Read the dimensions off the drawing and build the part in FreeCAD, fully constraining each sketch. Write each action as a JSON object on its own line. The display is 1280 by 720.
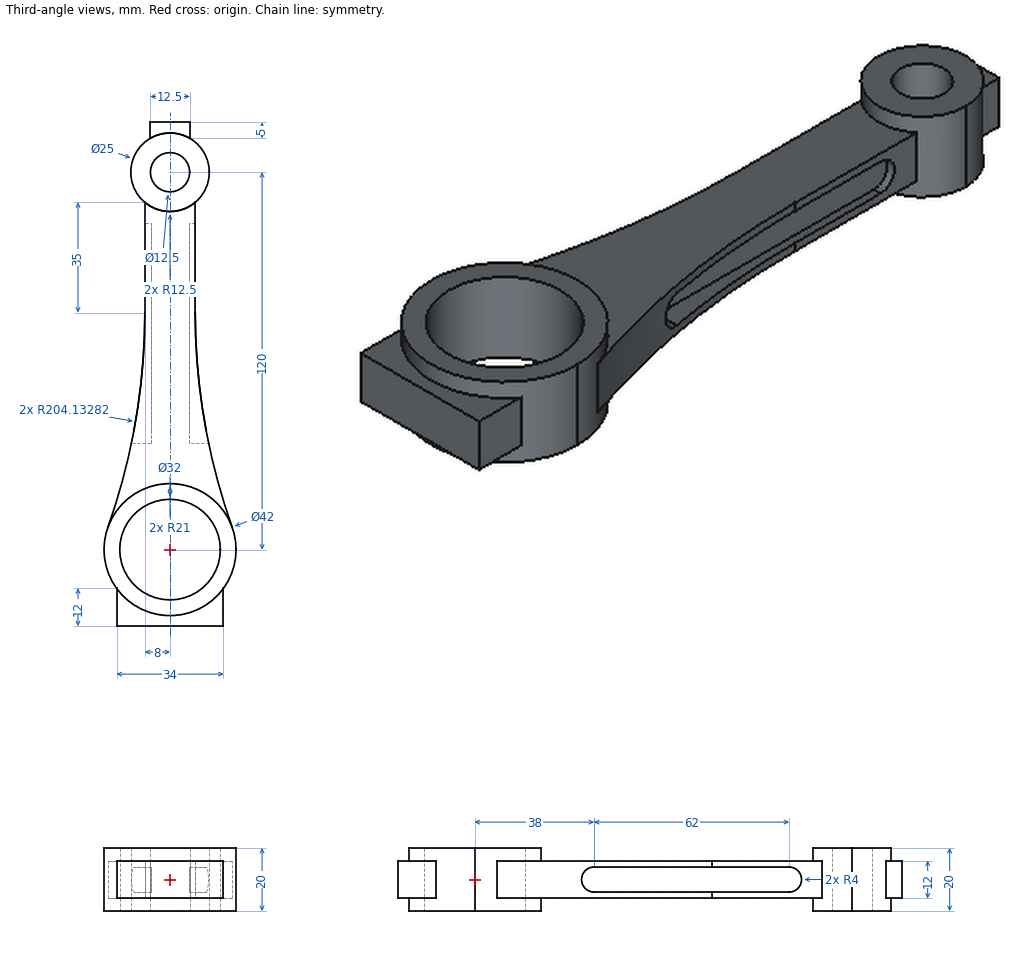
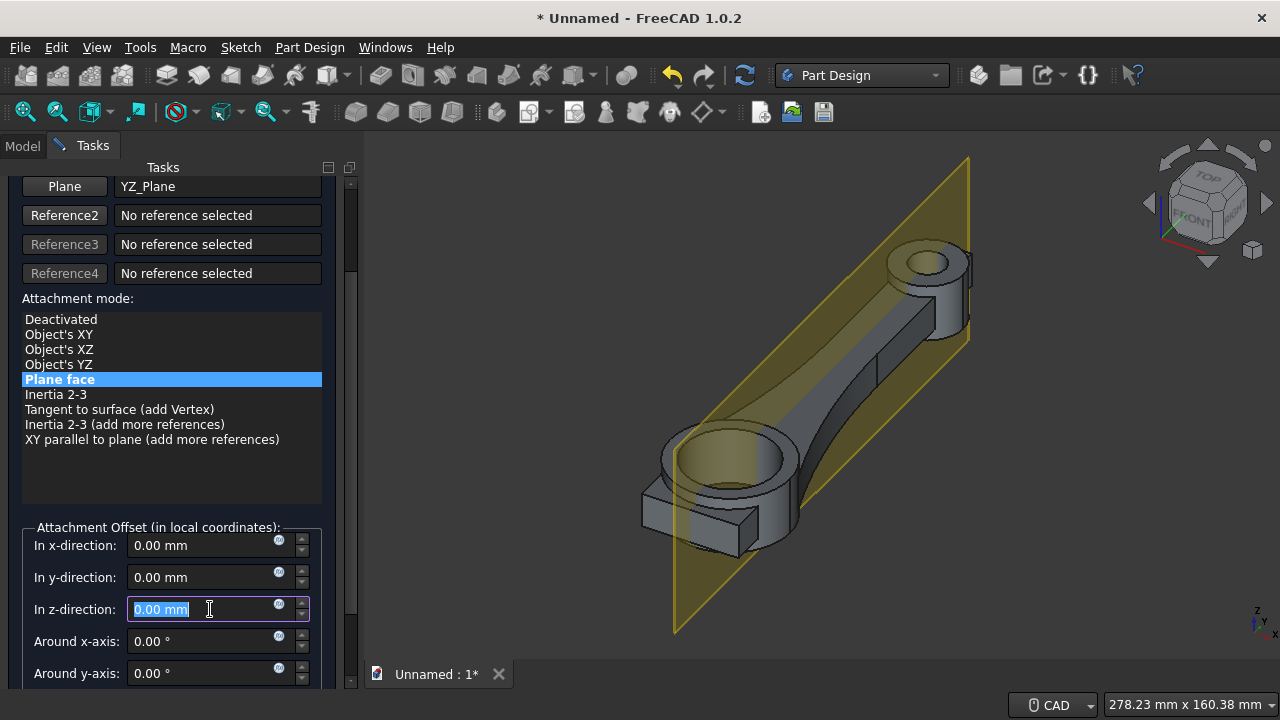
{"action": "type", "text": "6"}
{"action": "key", "text": "Tab"}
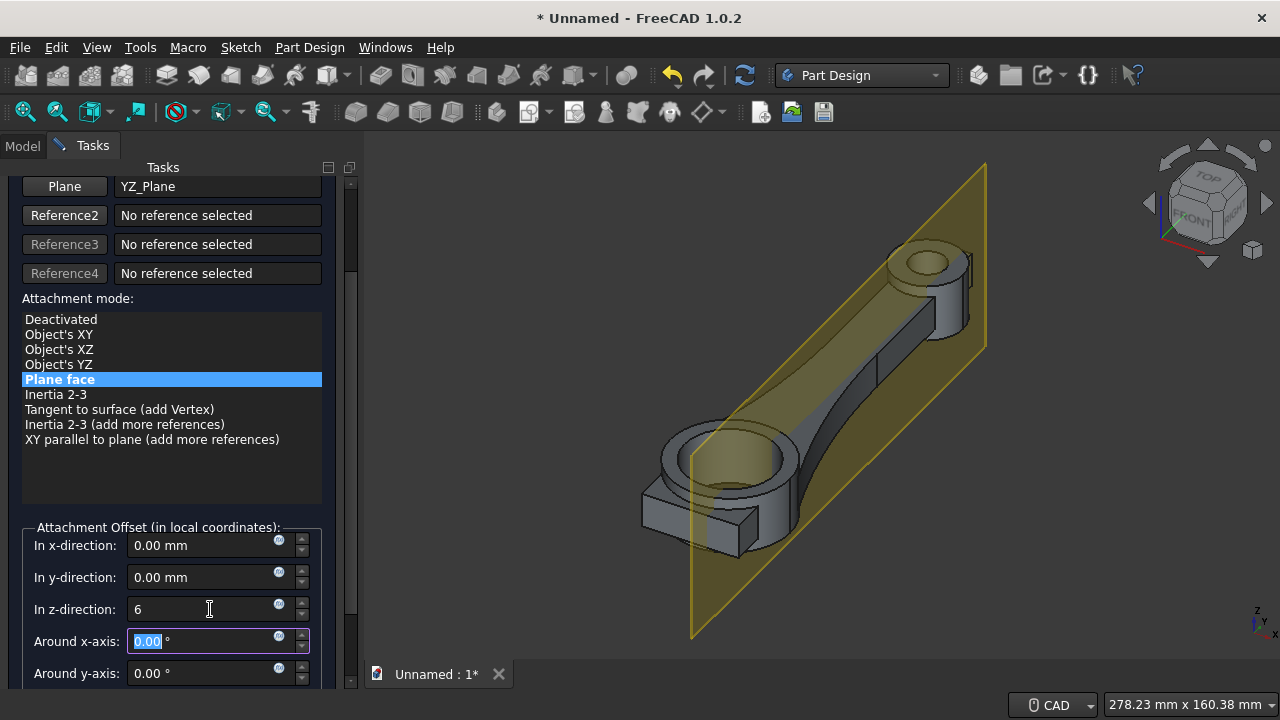
{"action": "scroll", "coordinate": [351, 432], "scroll_direction": "up", "scroll_amount": 3}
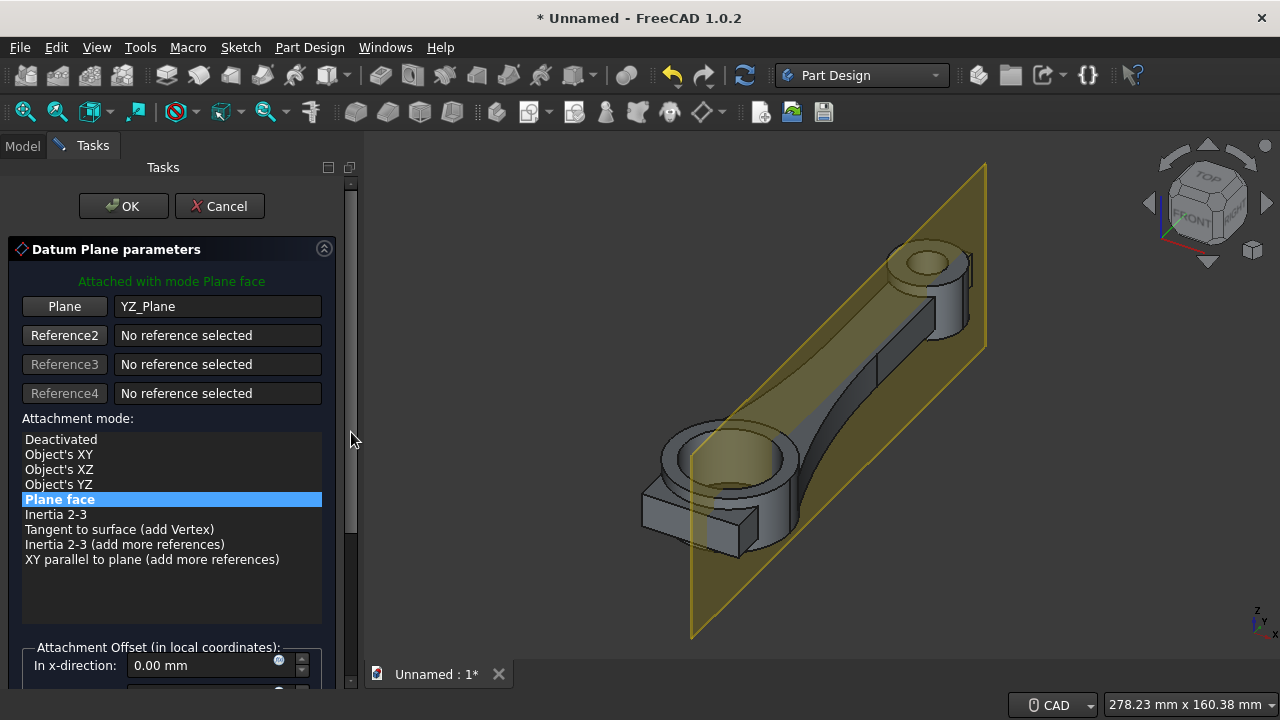
{"action": "left_click", "coordinate": [124, 206]}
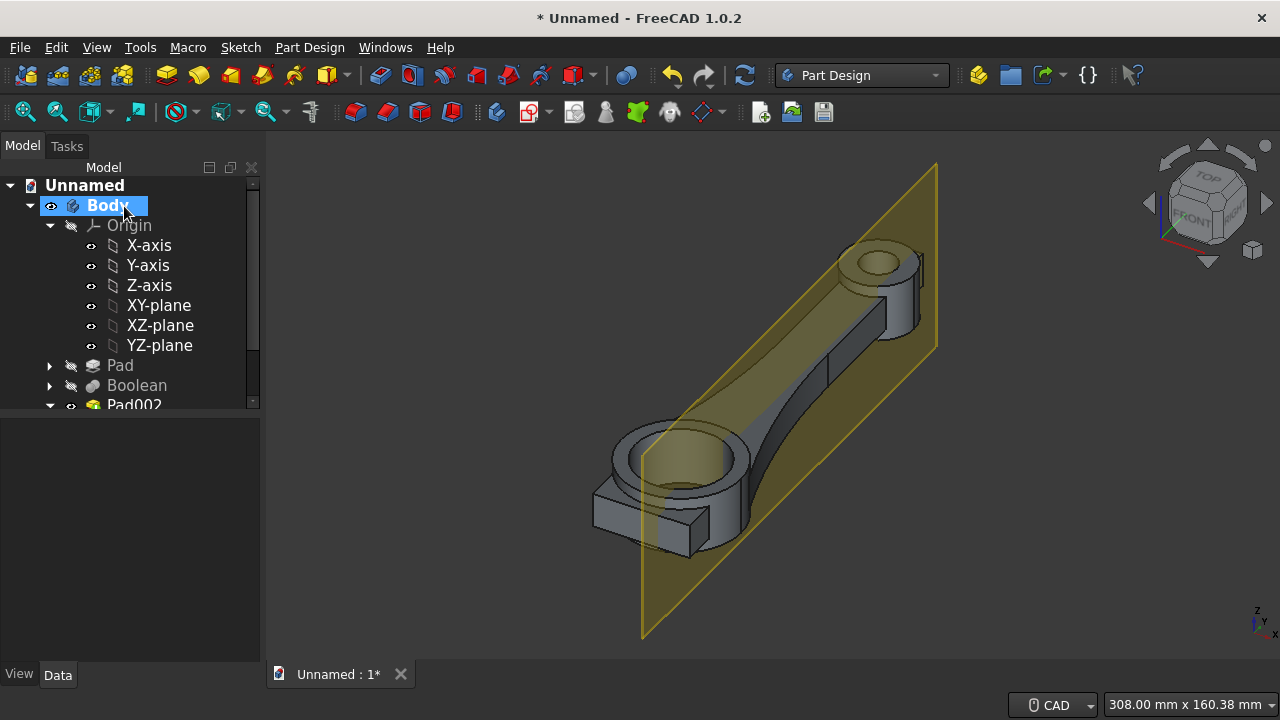
{"action": "scroll", "coordinate": [100, 301], "scroll_direction": "down", "scroll_amount": 3}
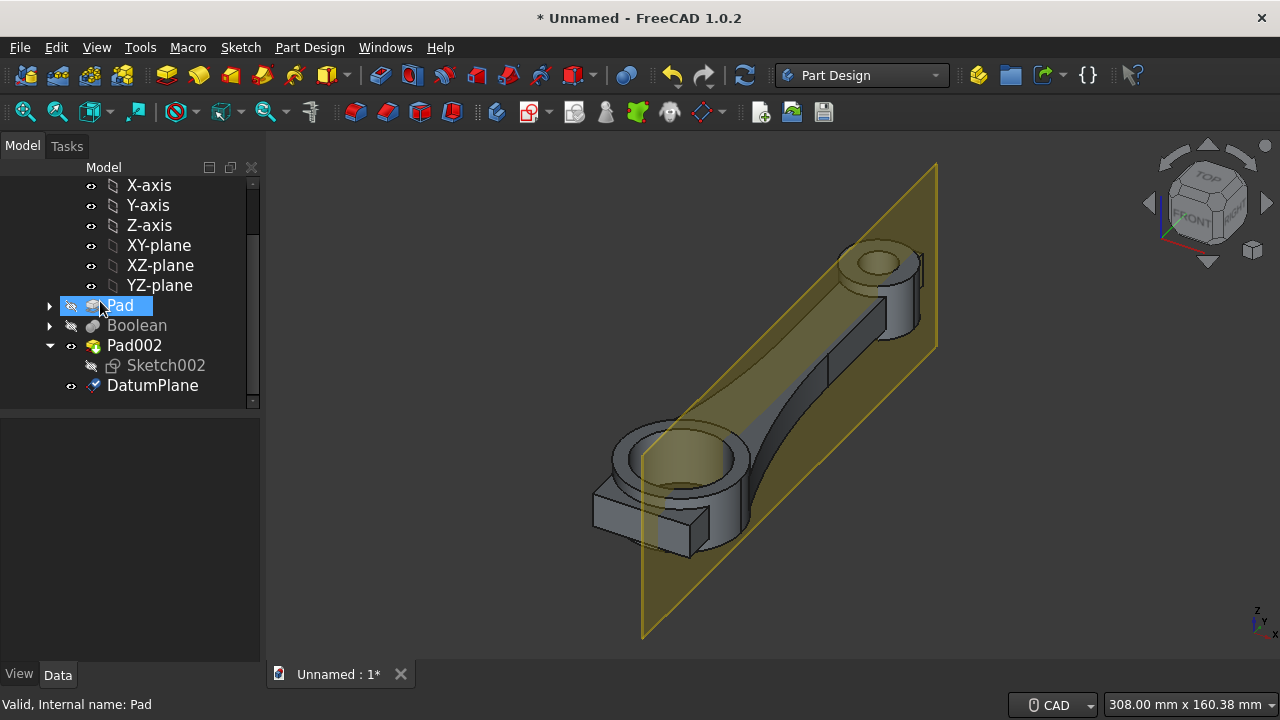
{"action": "left_click", "coordinate": [116, 386]}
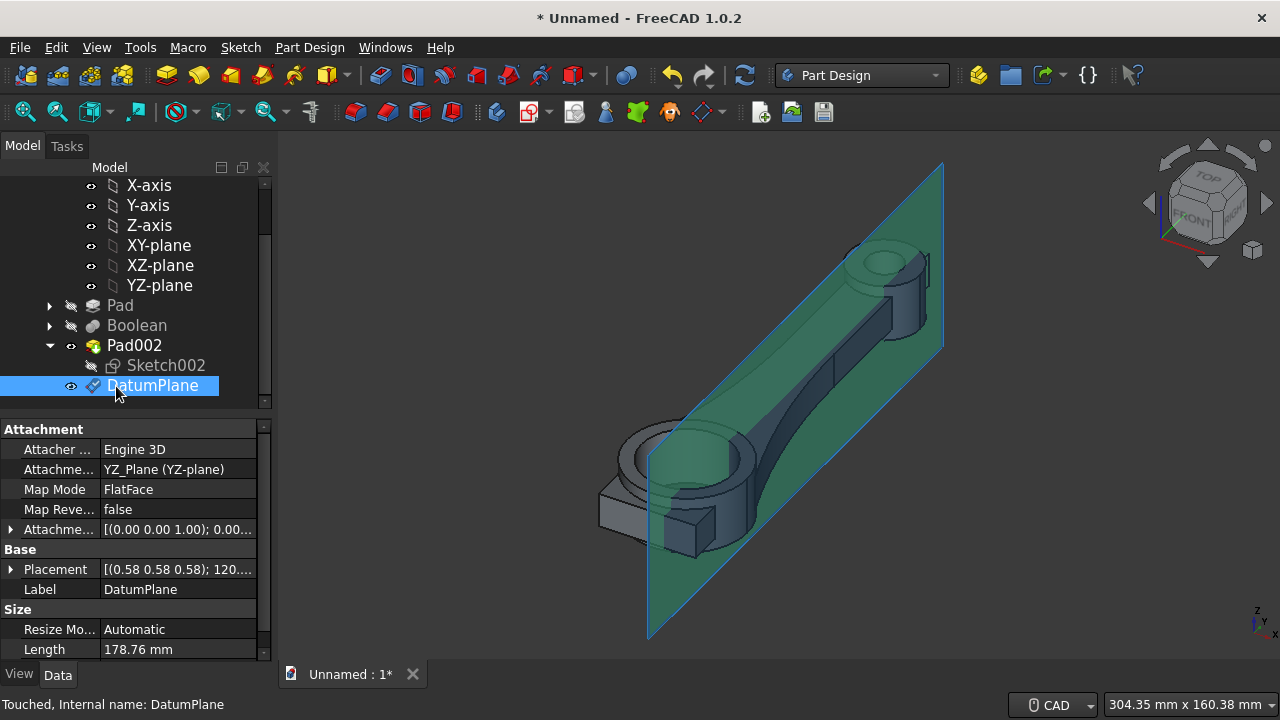
{"action": "left_click", "coordinate": [530, 112]}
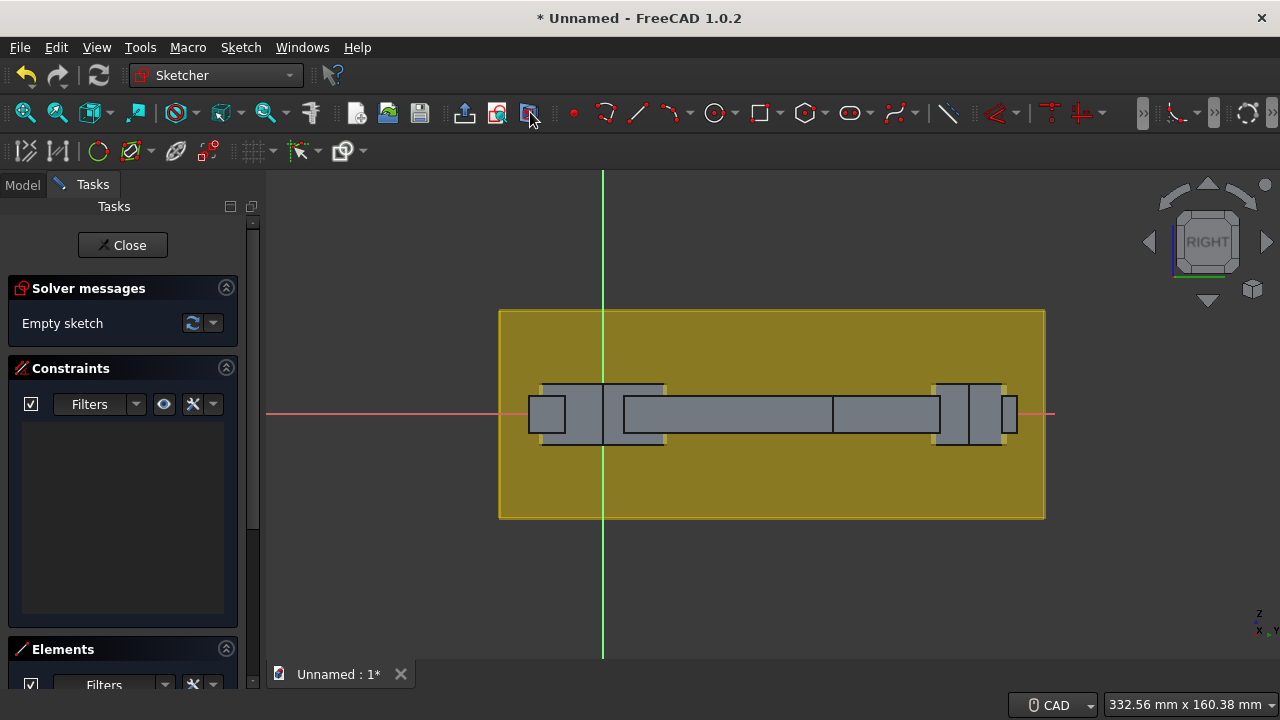
{"action": "key", "text": "q s"}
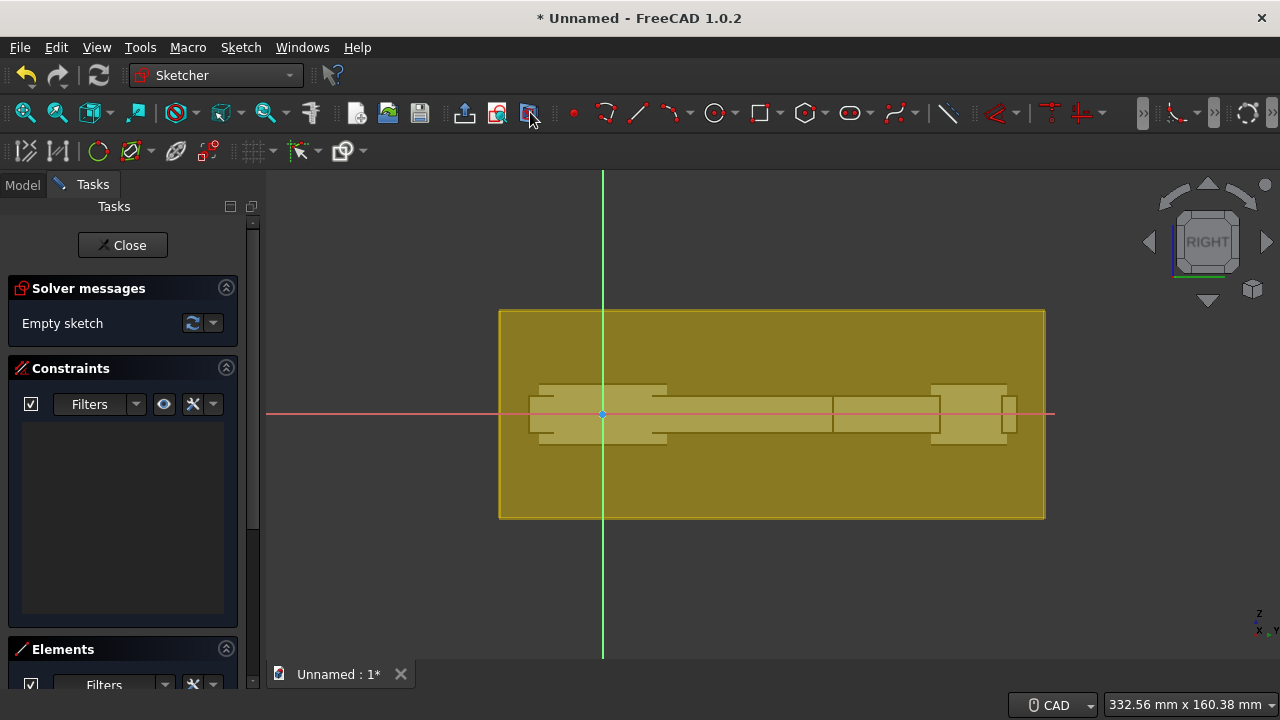
{"action": "scroll", "coordinate": [831, 414], "scroll_direction": "up", "scroll_amount": 3}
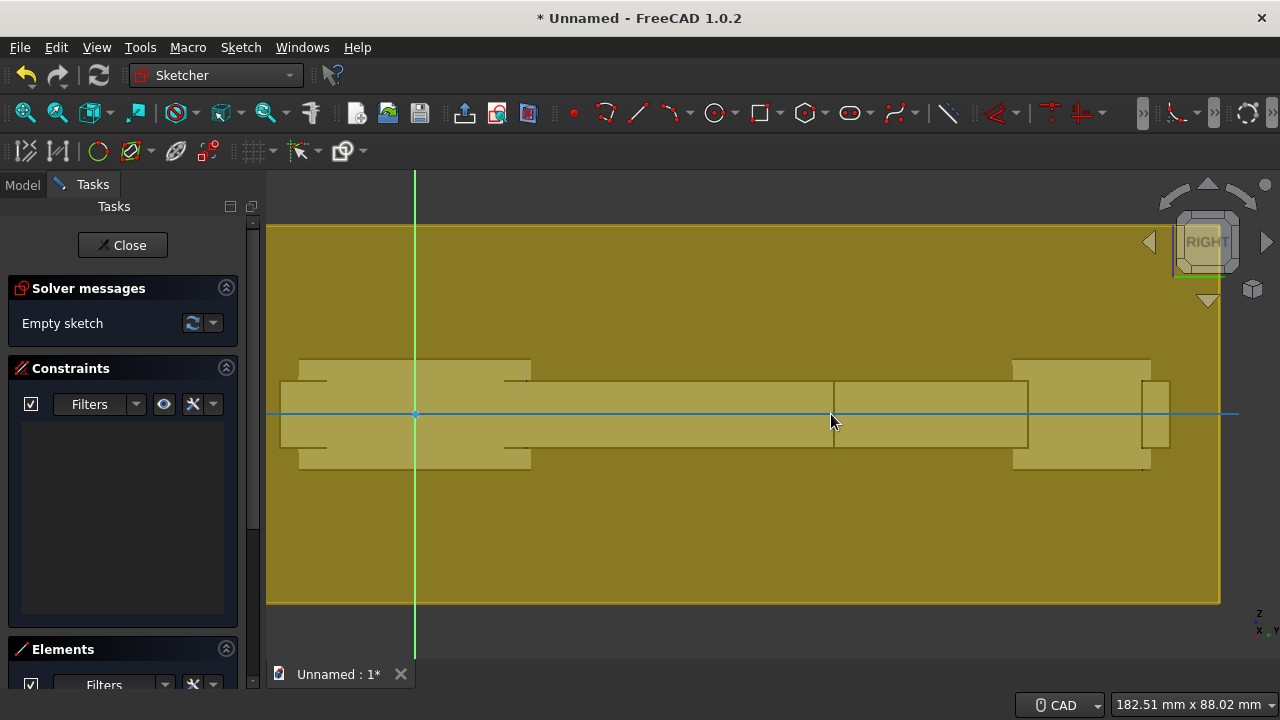
{"action": "key", "text": "g s"}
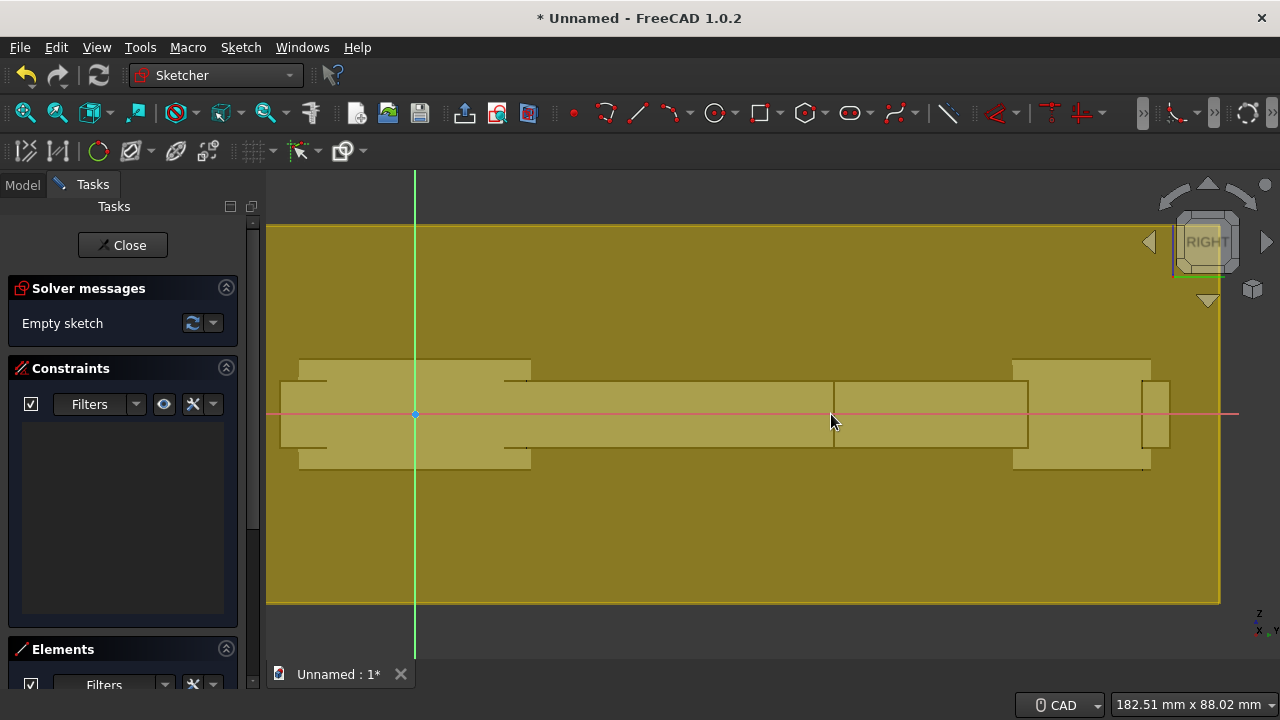
{"action": "left_click", "coordinate": [626, 414]}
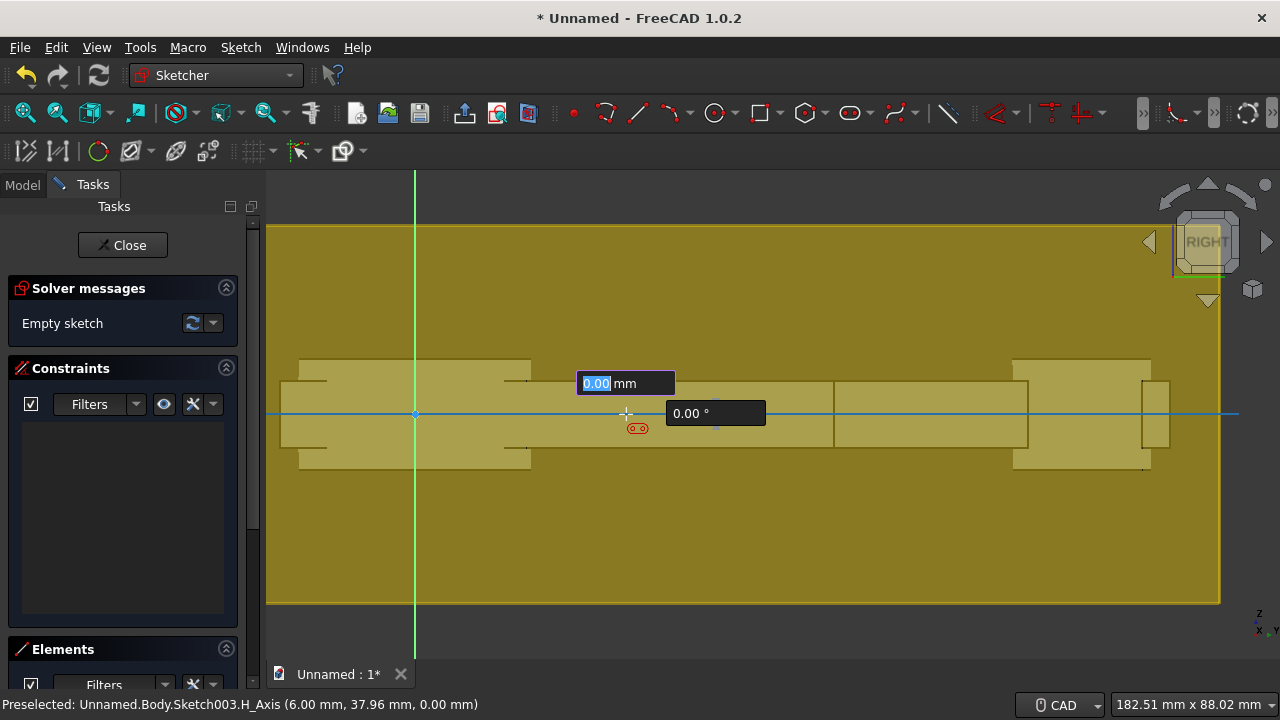
{"action": "left_click", "coordinate": [971, 405]}